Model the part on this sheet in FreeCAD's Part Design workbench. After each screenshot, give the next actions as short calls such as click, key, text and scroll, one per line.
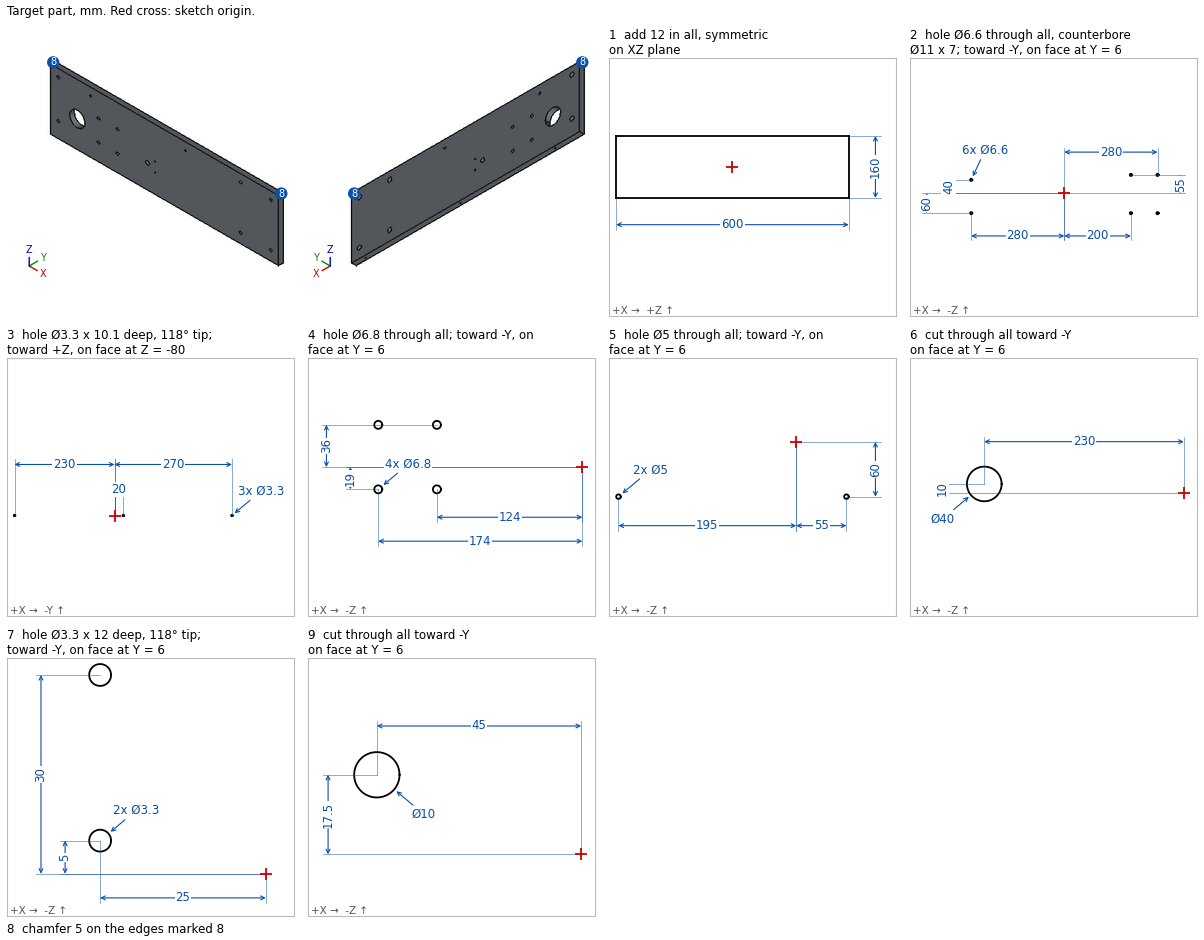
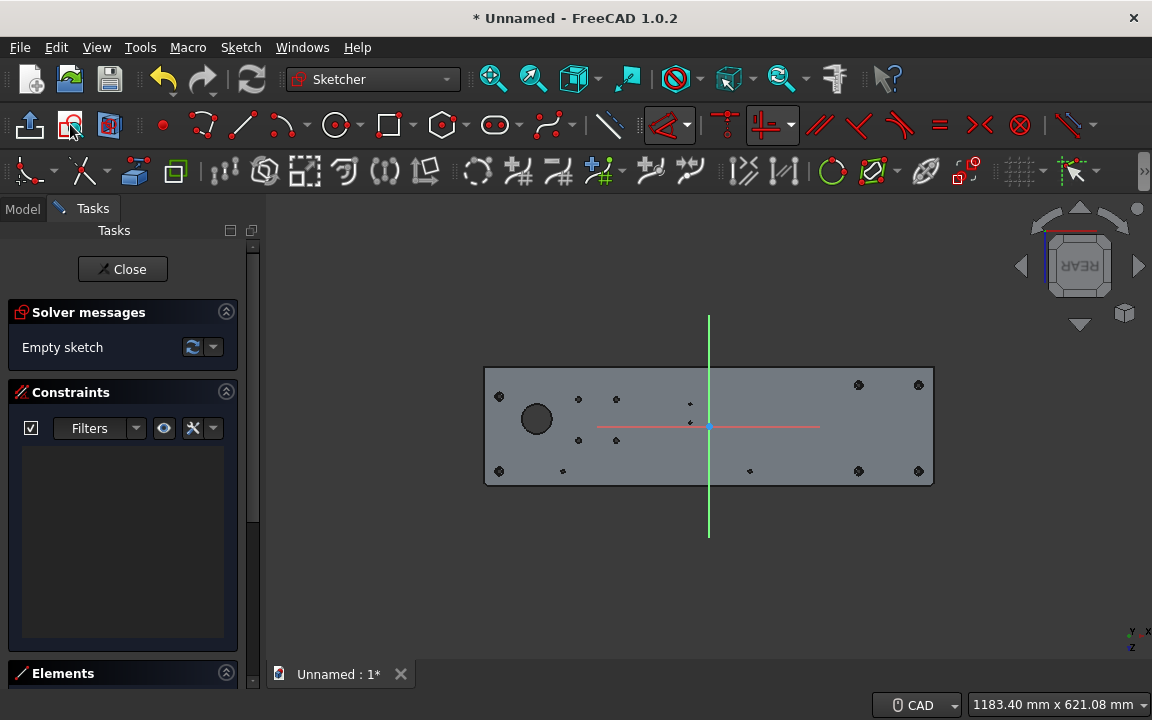
scroll(677, 413, up, 15)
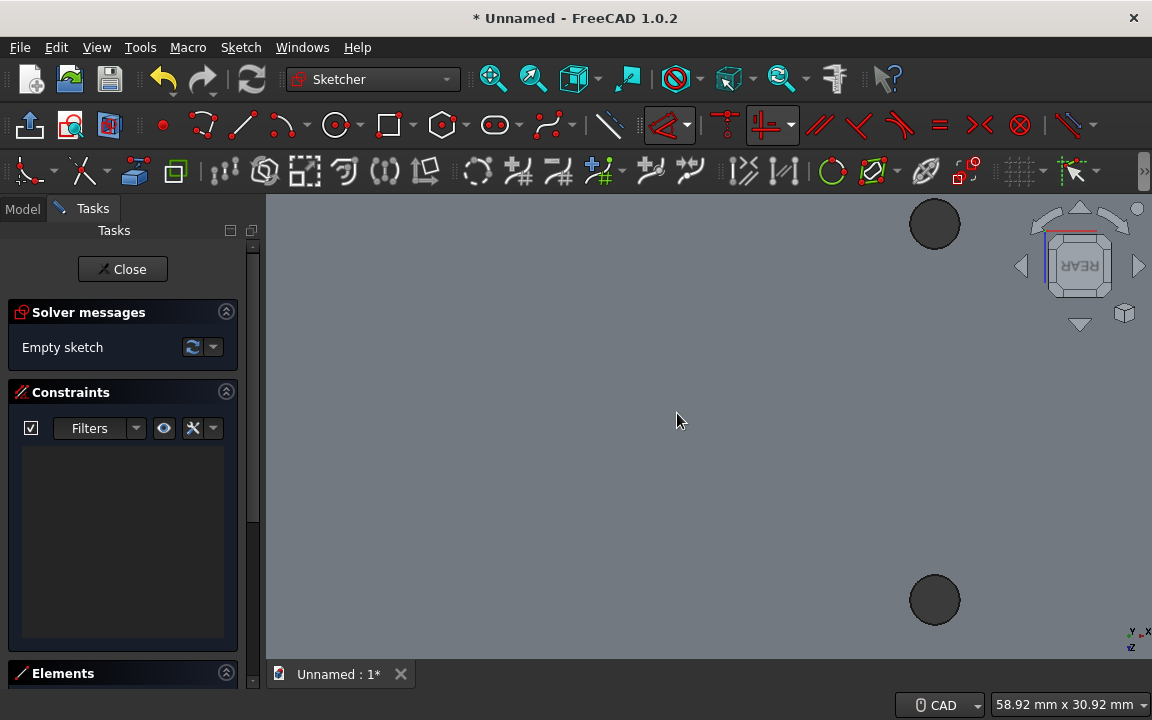
scroll(626, 394, up, 3)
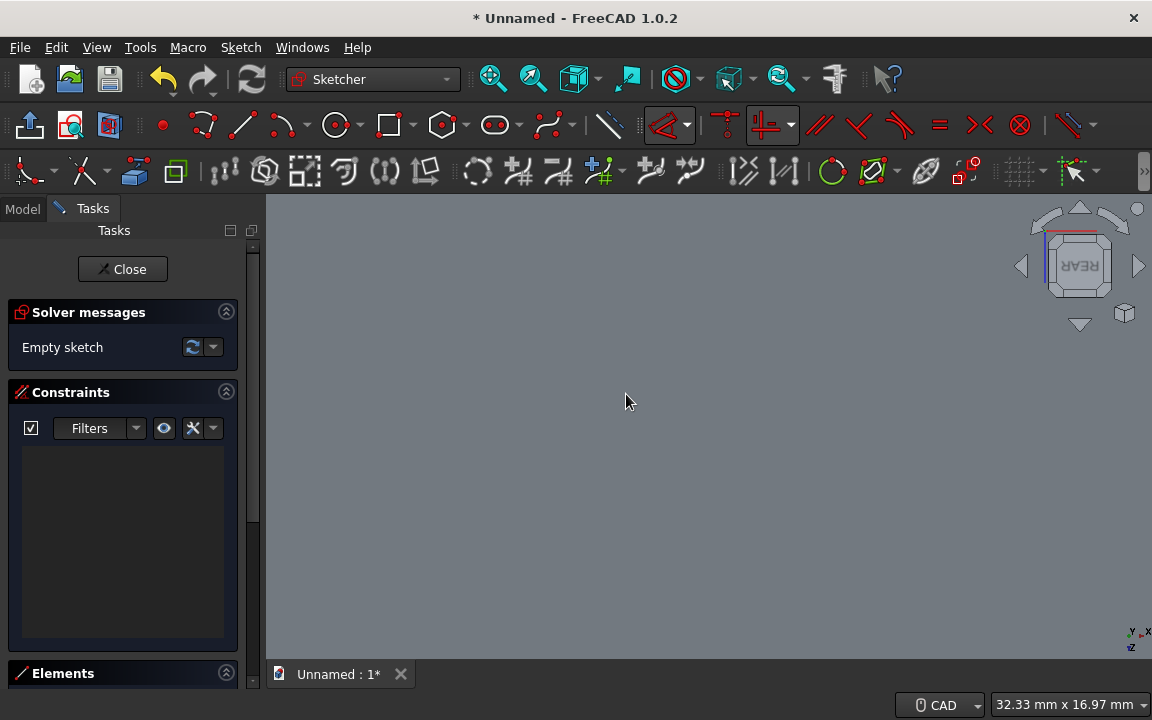
click(336, 126)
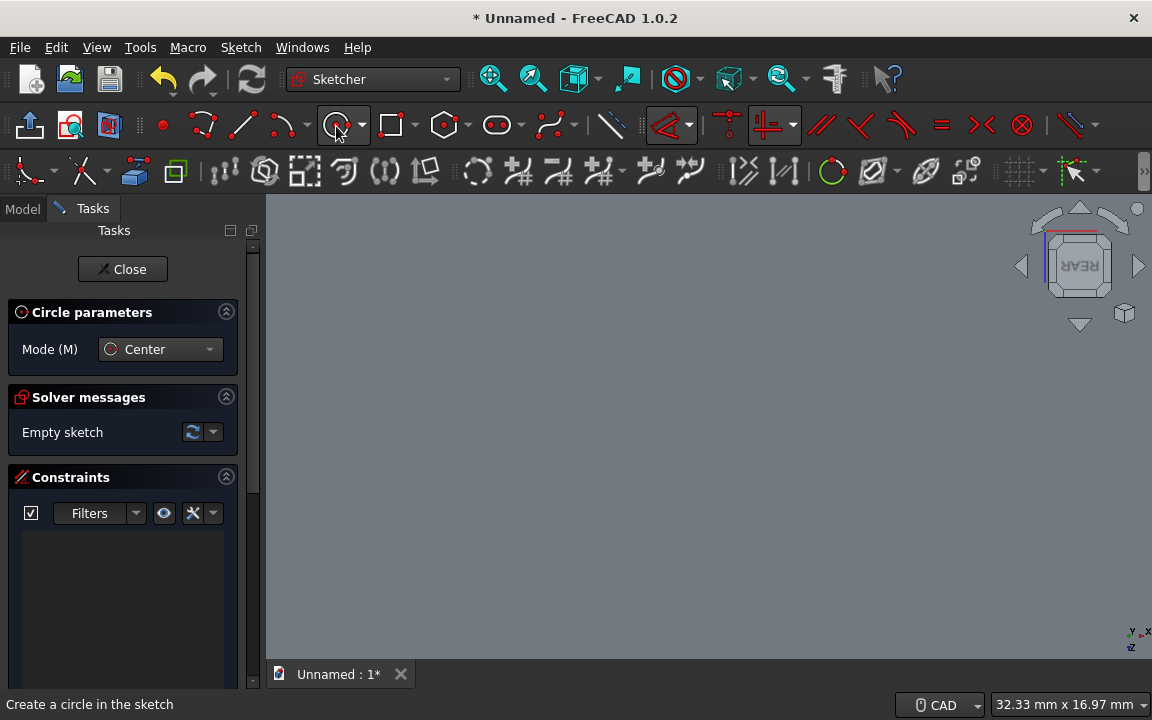
click(641, 426)
move(737, 330)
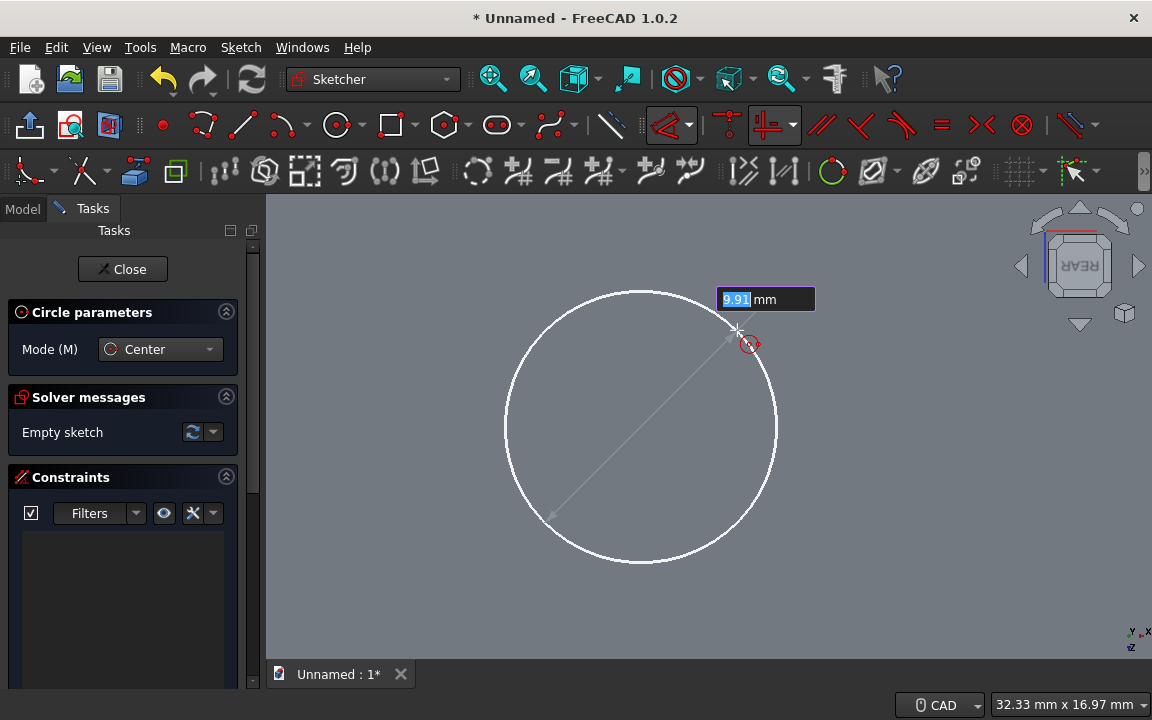
text(10)
key(Return)
key(Escape)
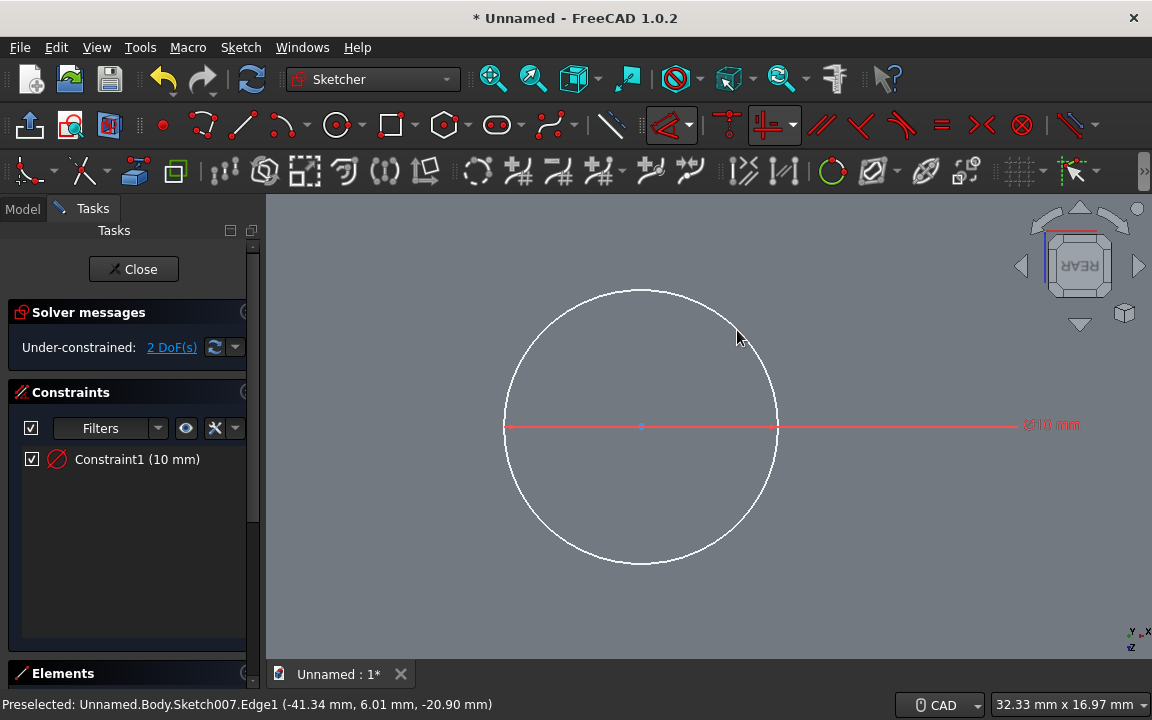
click(641, 427)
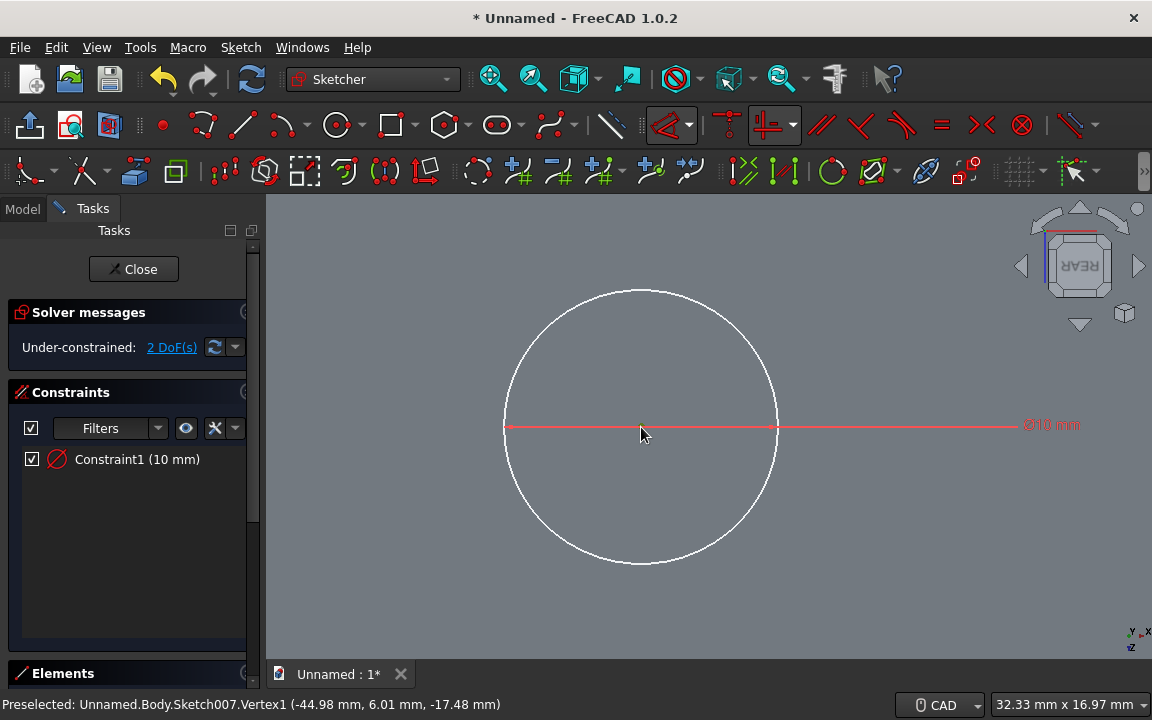
key(l)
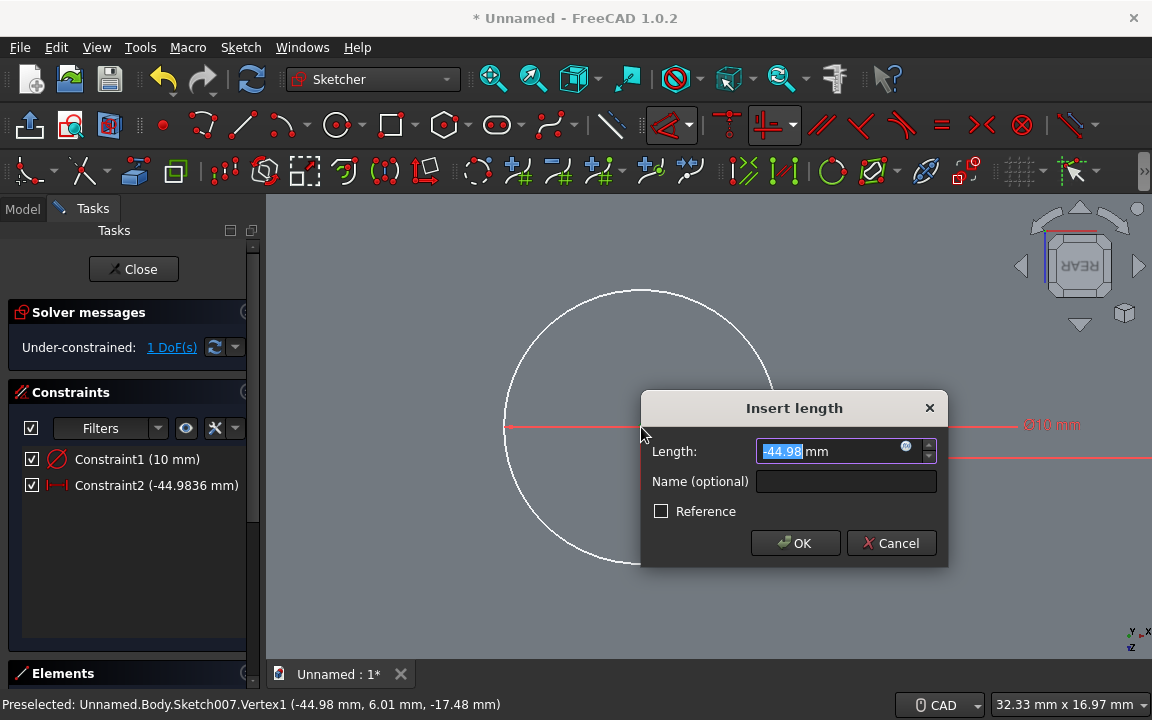
text(-45)
key(Return)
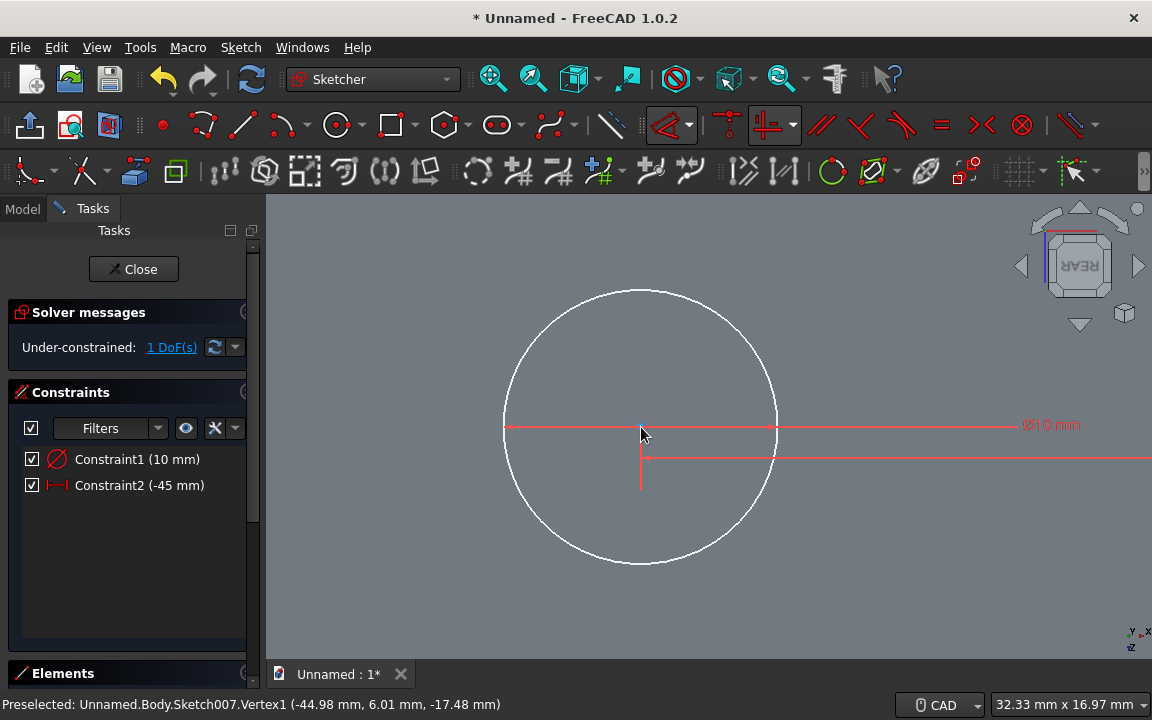
click(641, 427)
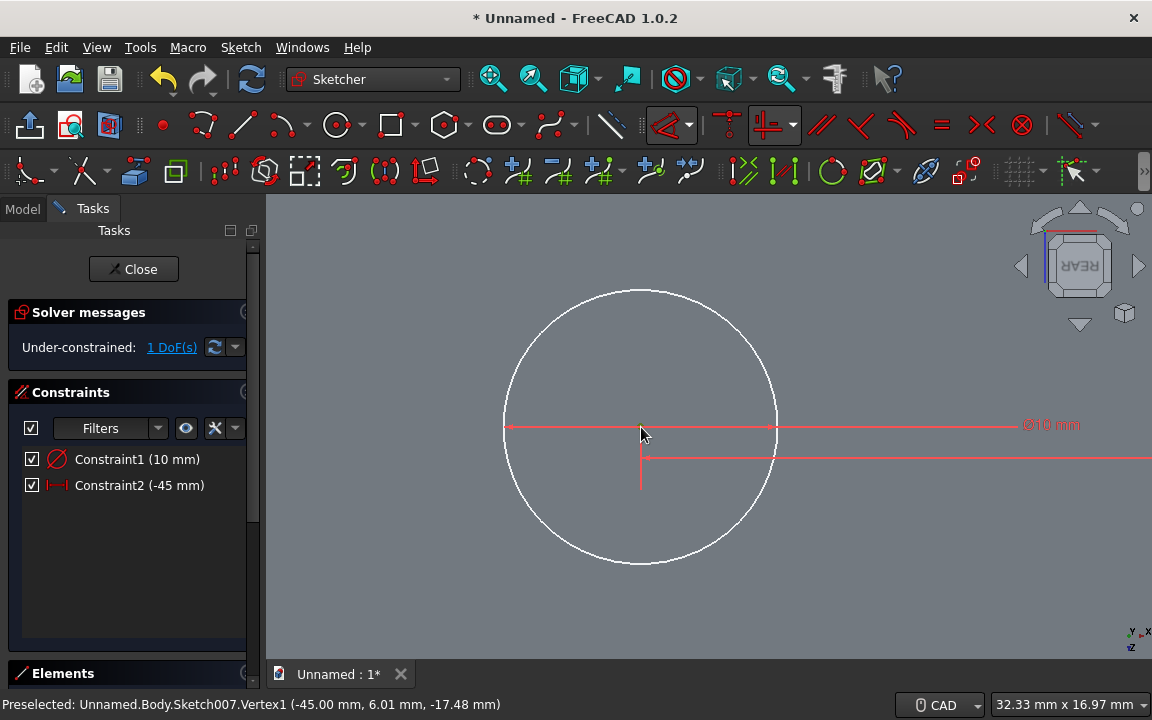
key(i)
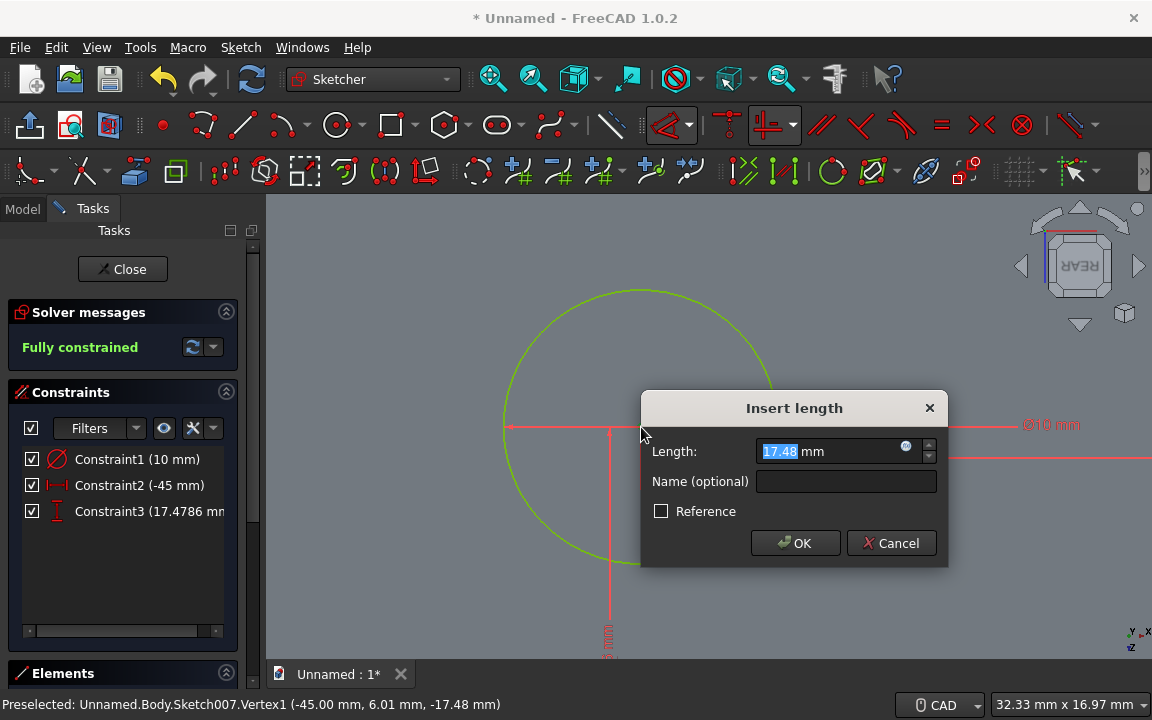
text(17.5)
key(Return)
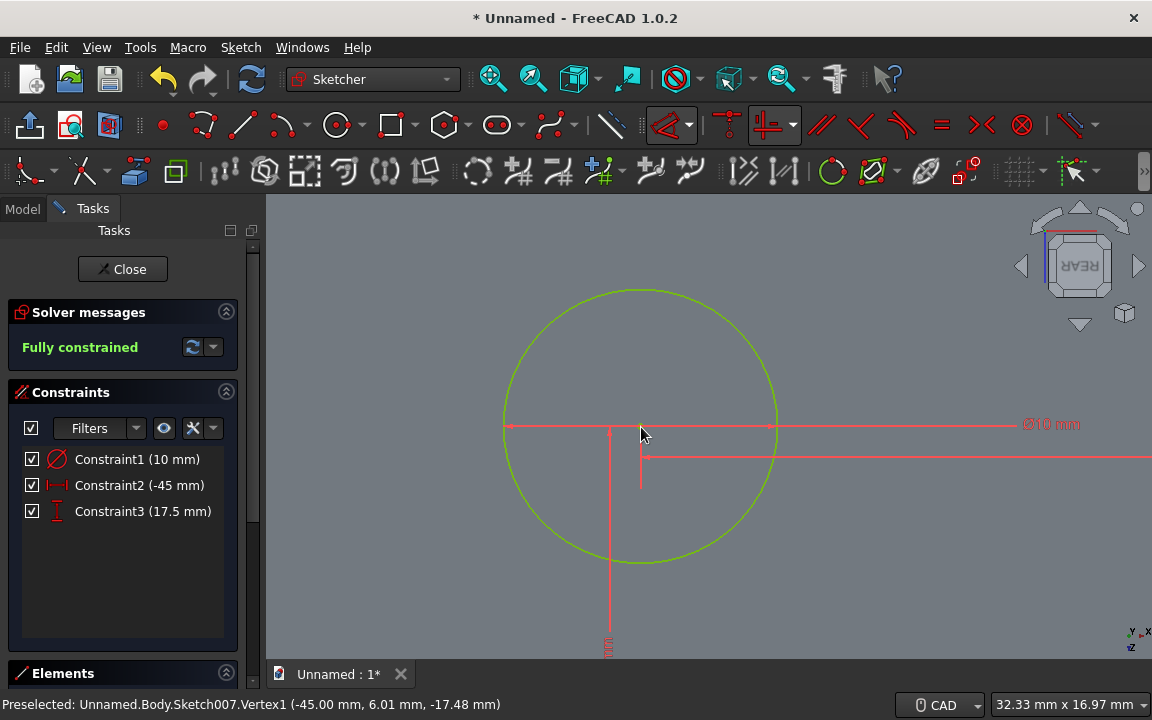
click(123, 269)